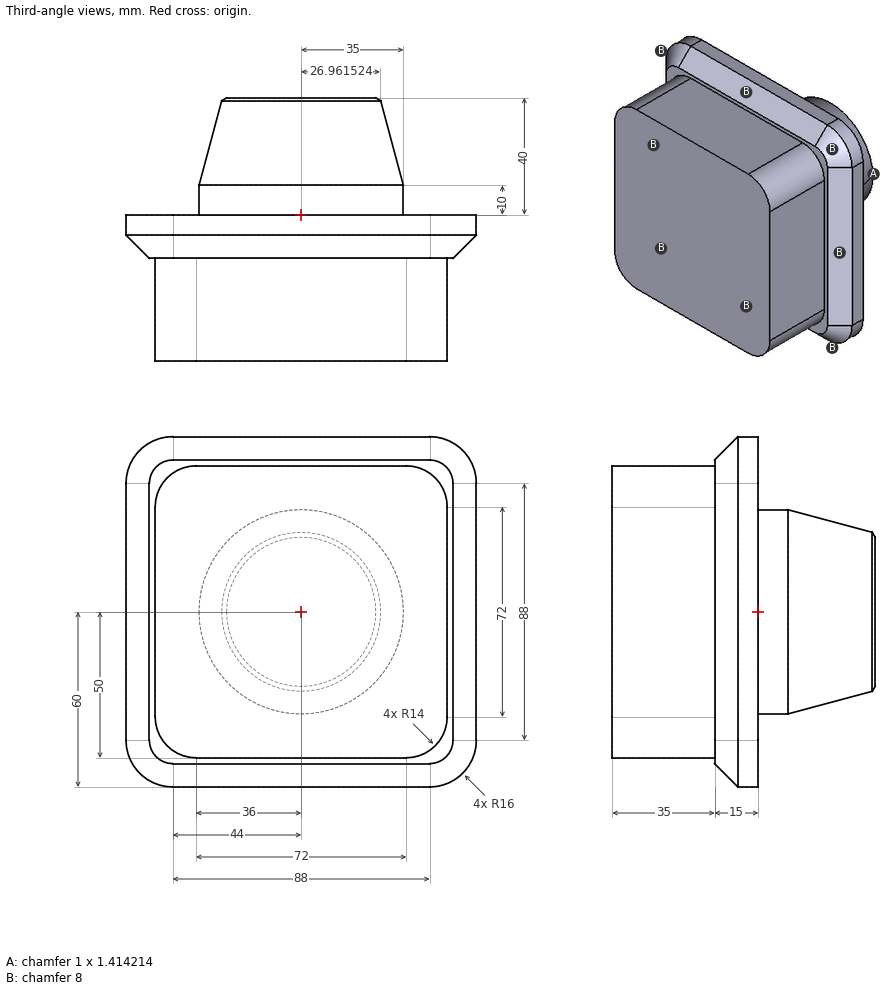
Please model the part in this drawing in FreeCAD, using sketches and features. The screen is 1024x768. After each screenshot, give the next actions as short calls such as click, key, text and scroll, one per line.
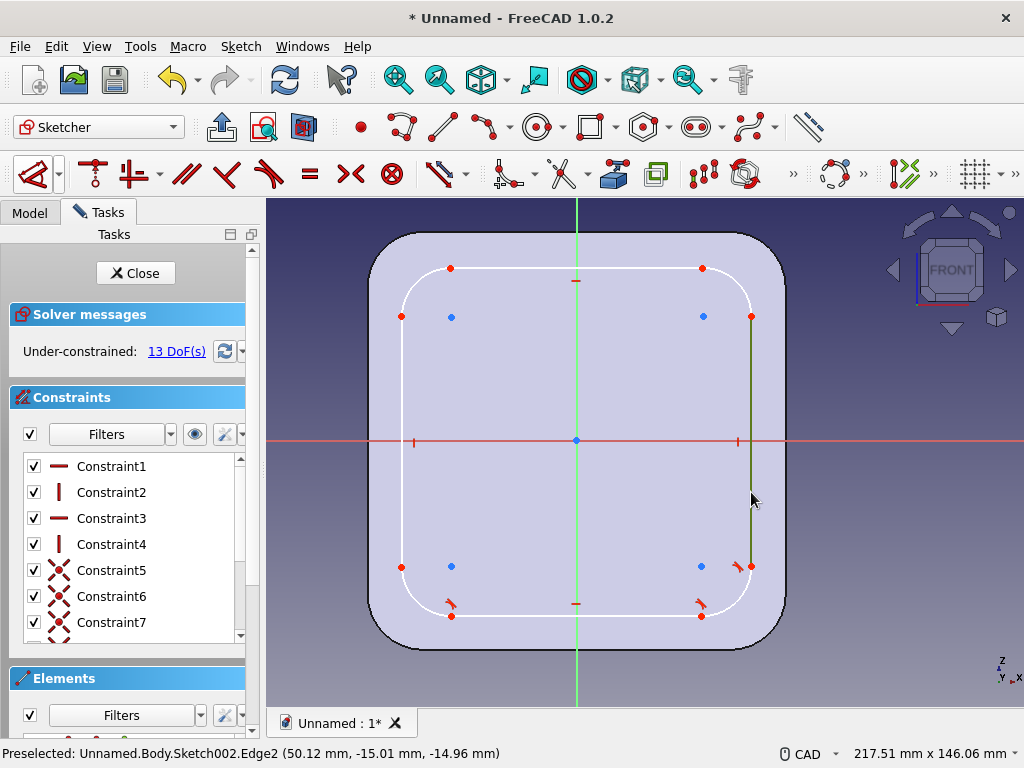
click(746, 295)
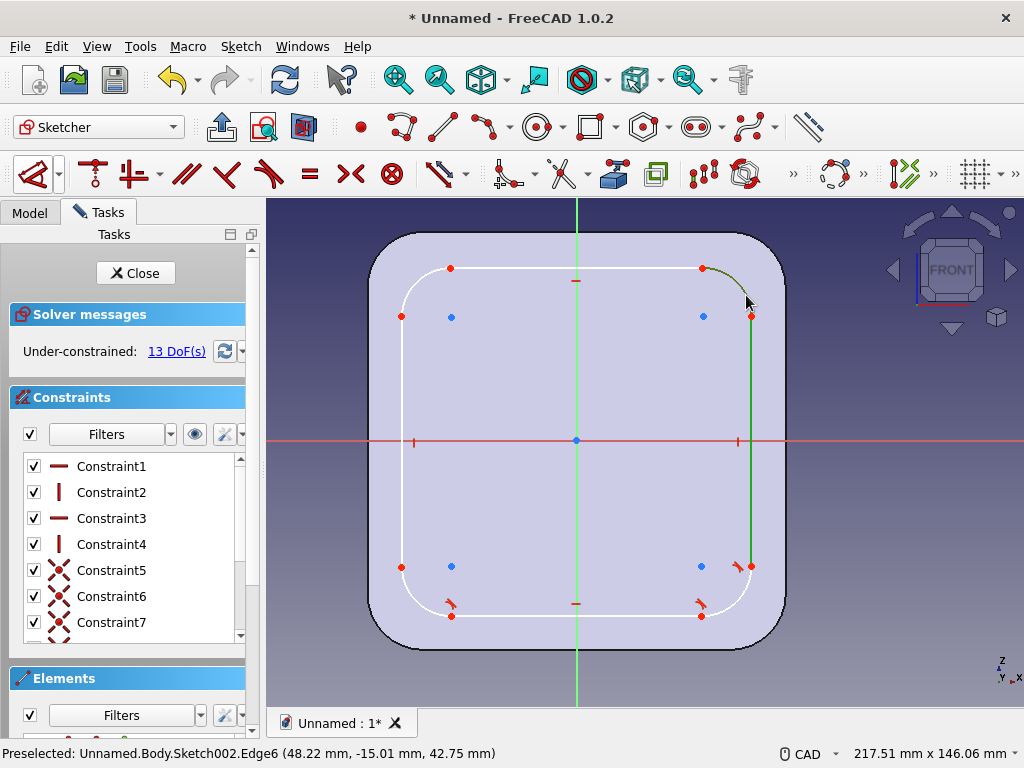
key(t)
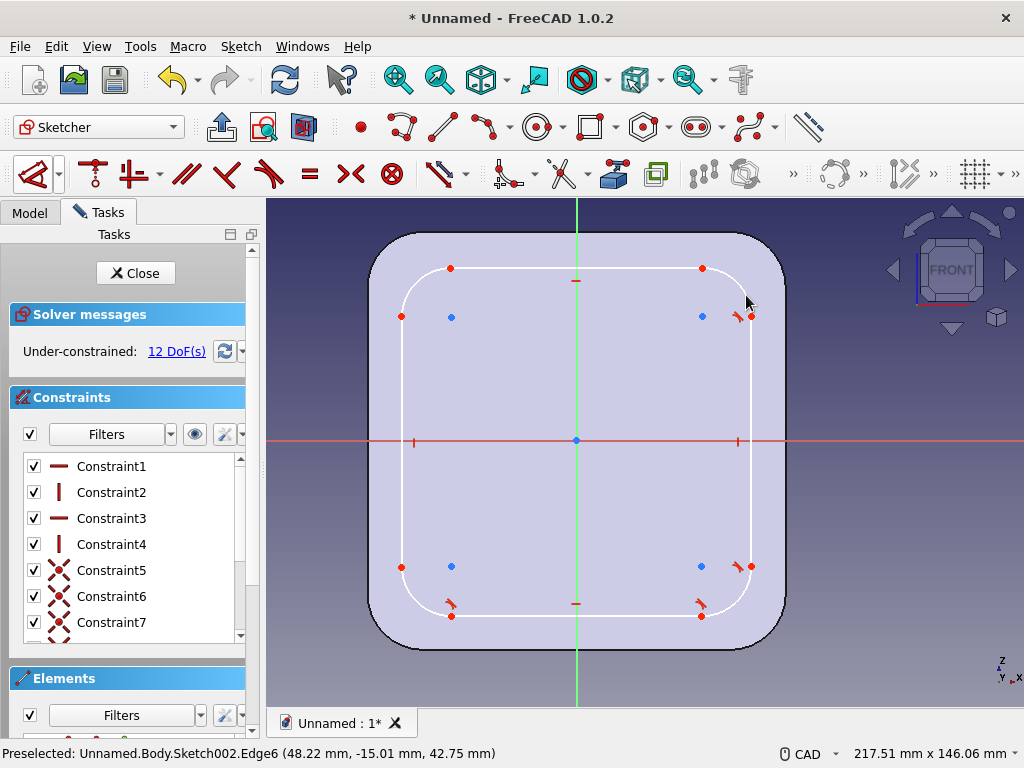
click(627, 268)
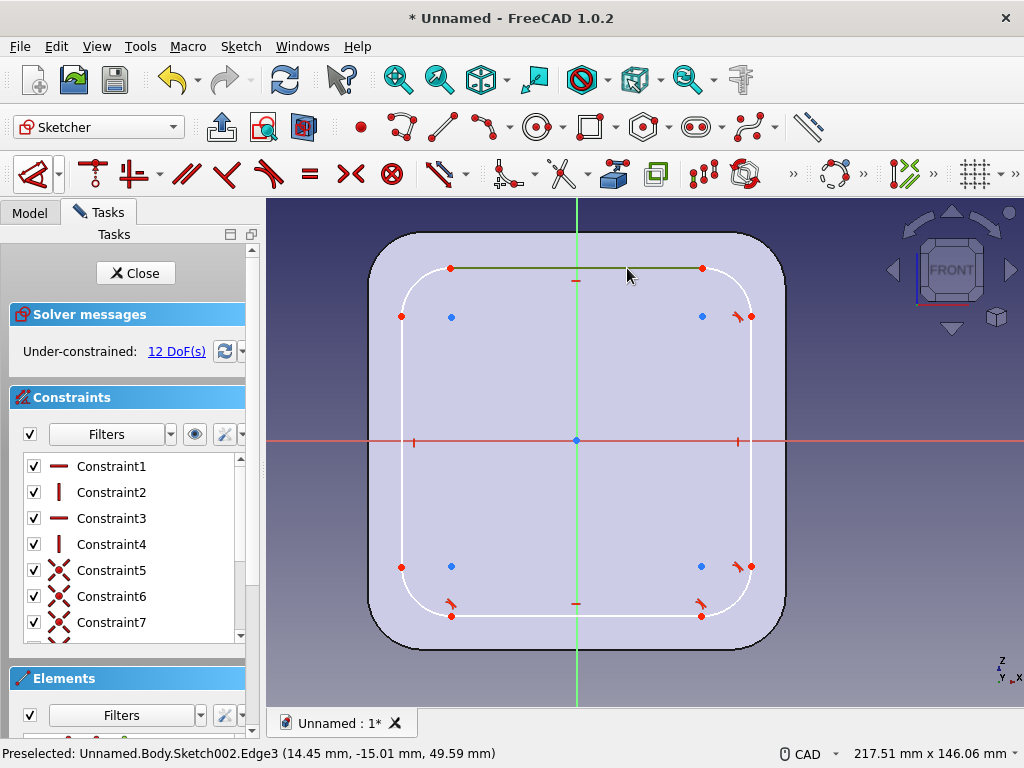
click(746, 295)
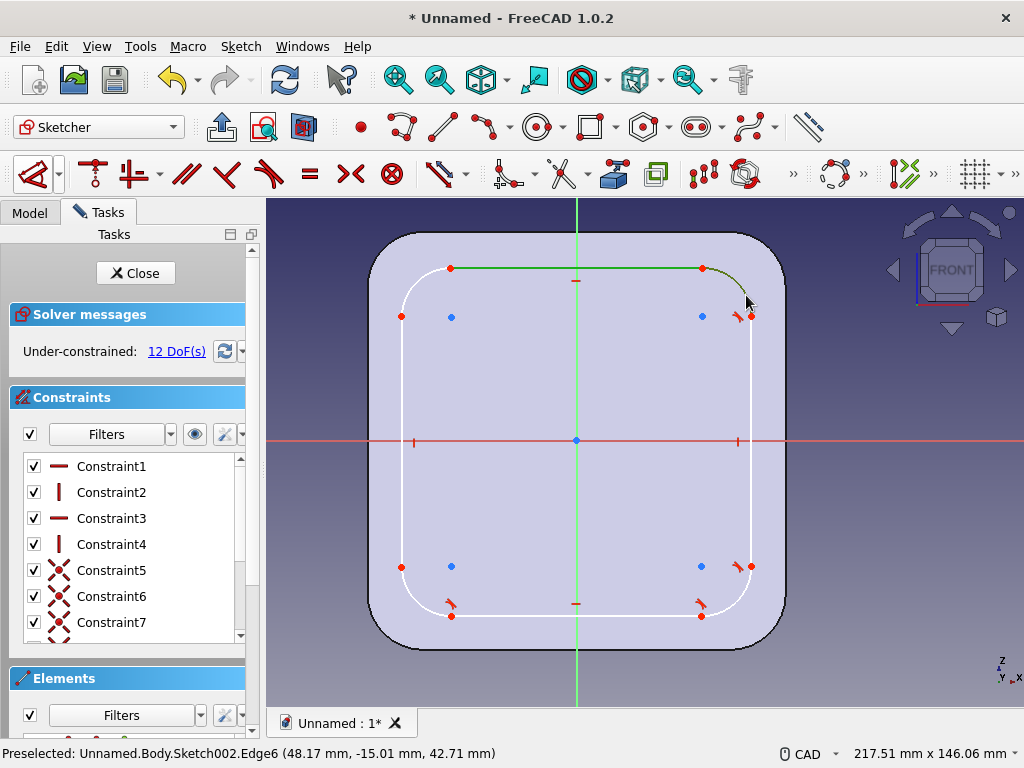
click(269, 174)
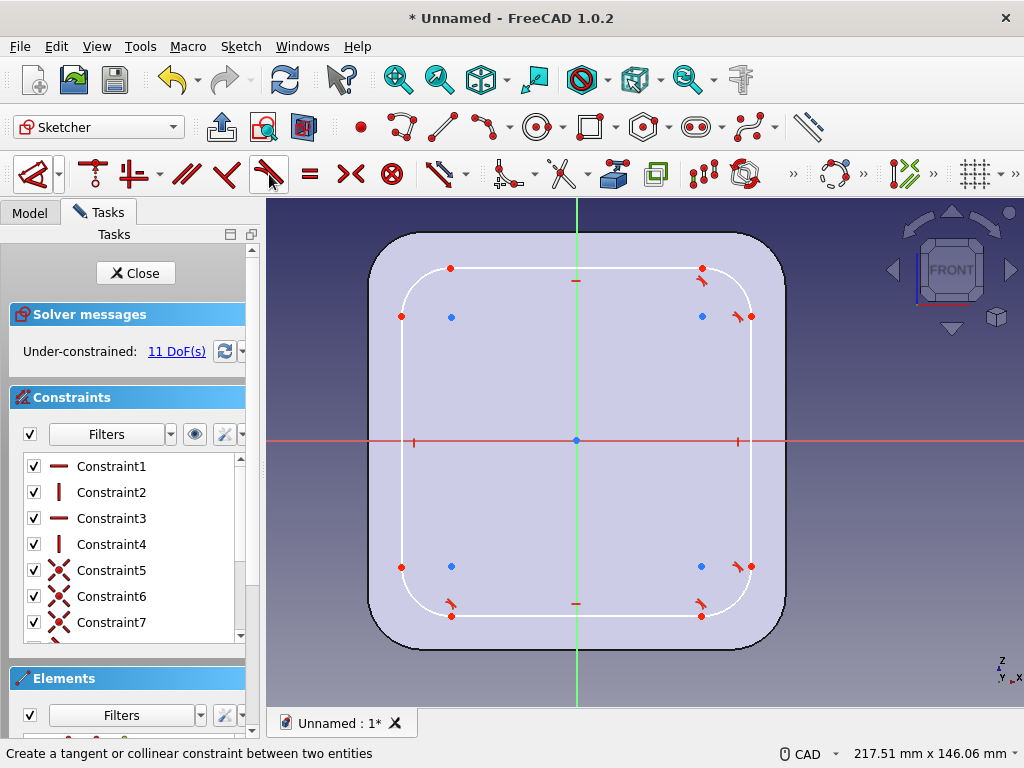
click(627, 268)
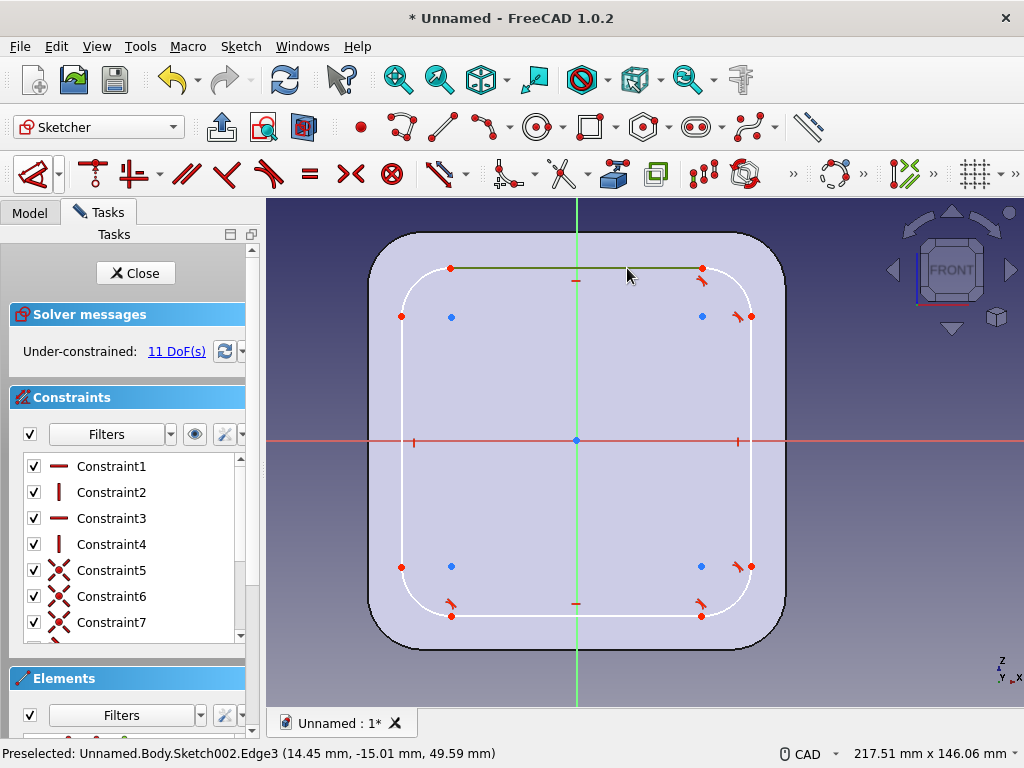
click(429, 274)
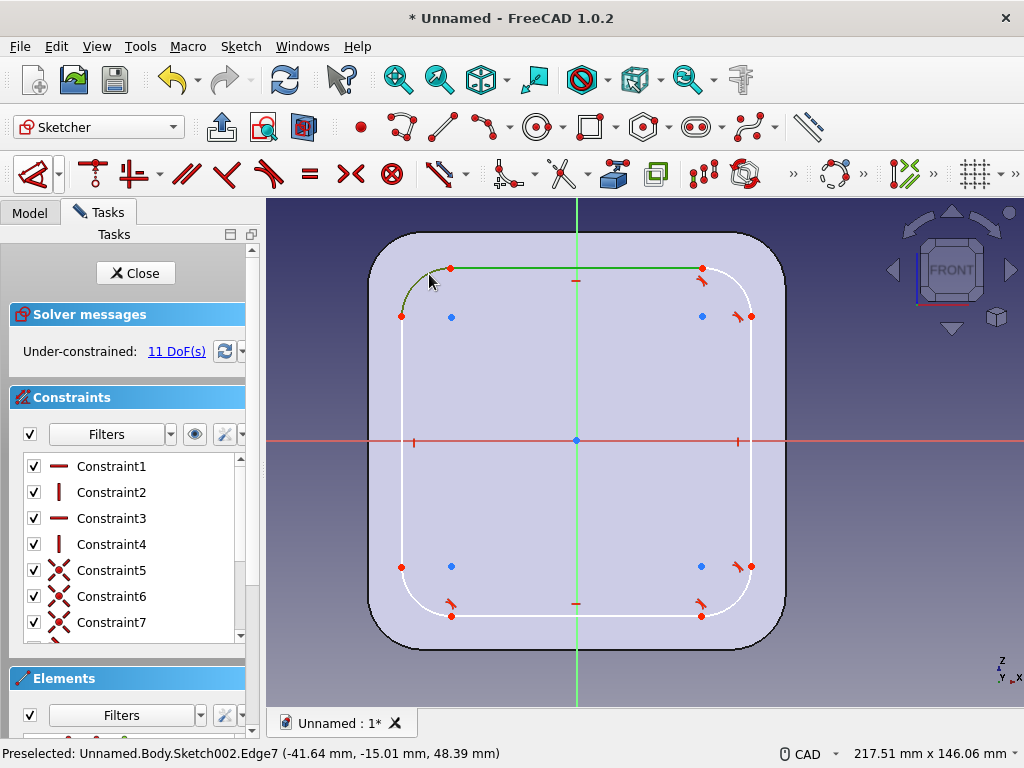
key(t)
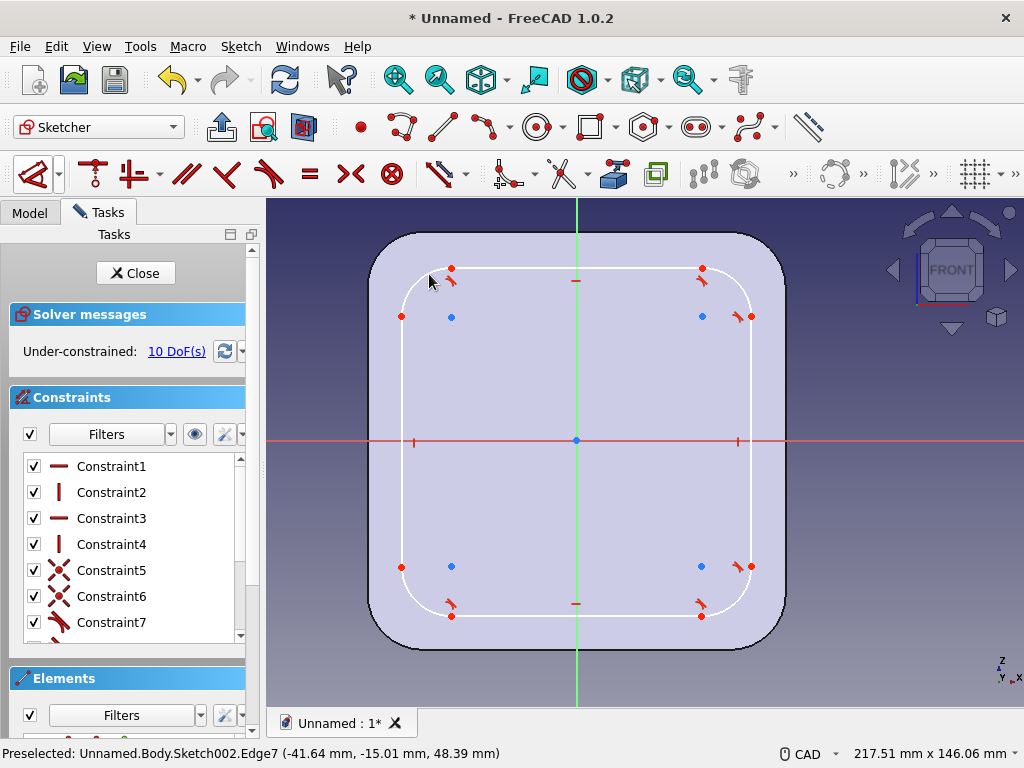
click(402, 392)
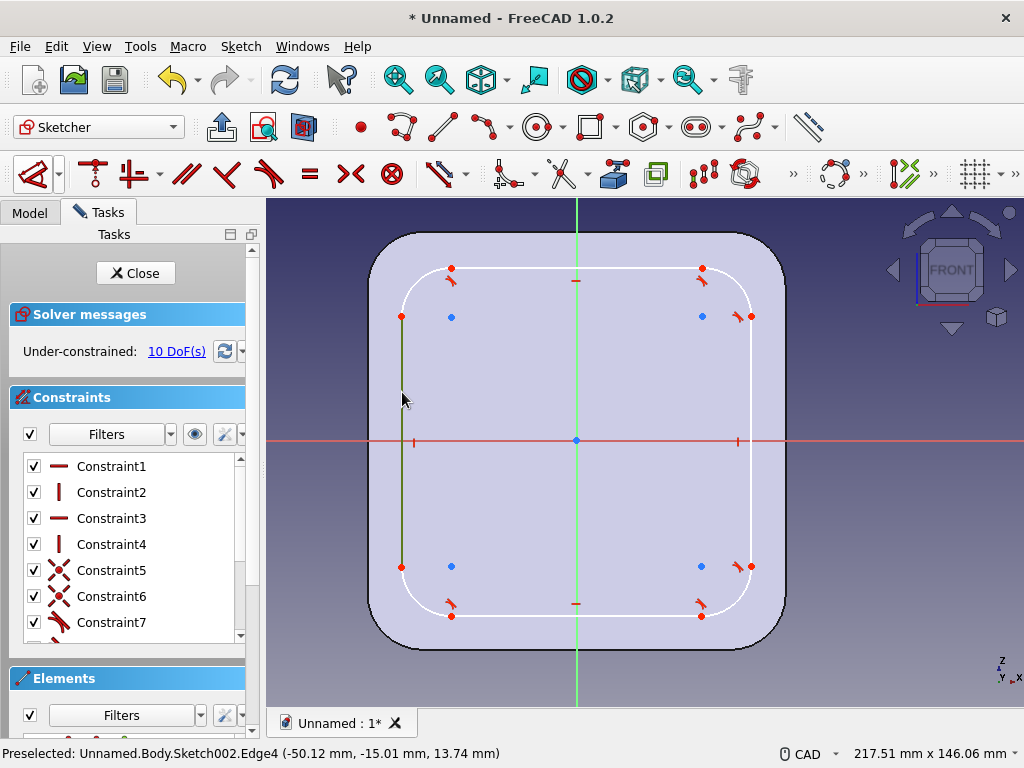
click(429, 273)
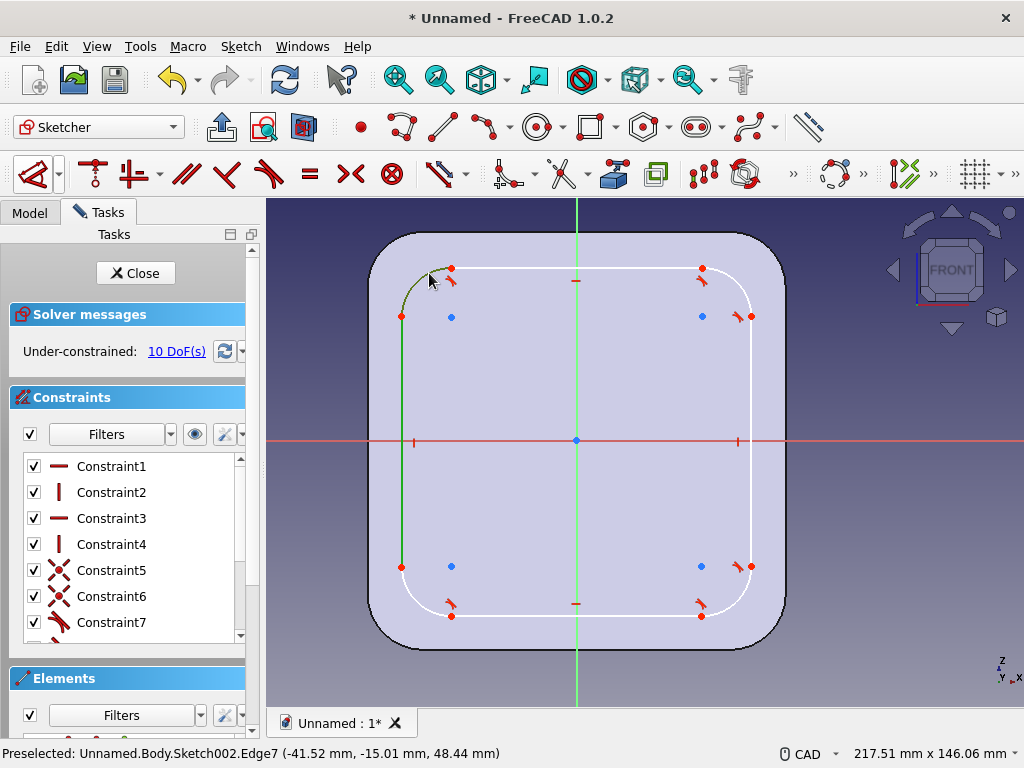
click(269, 174)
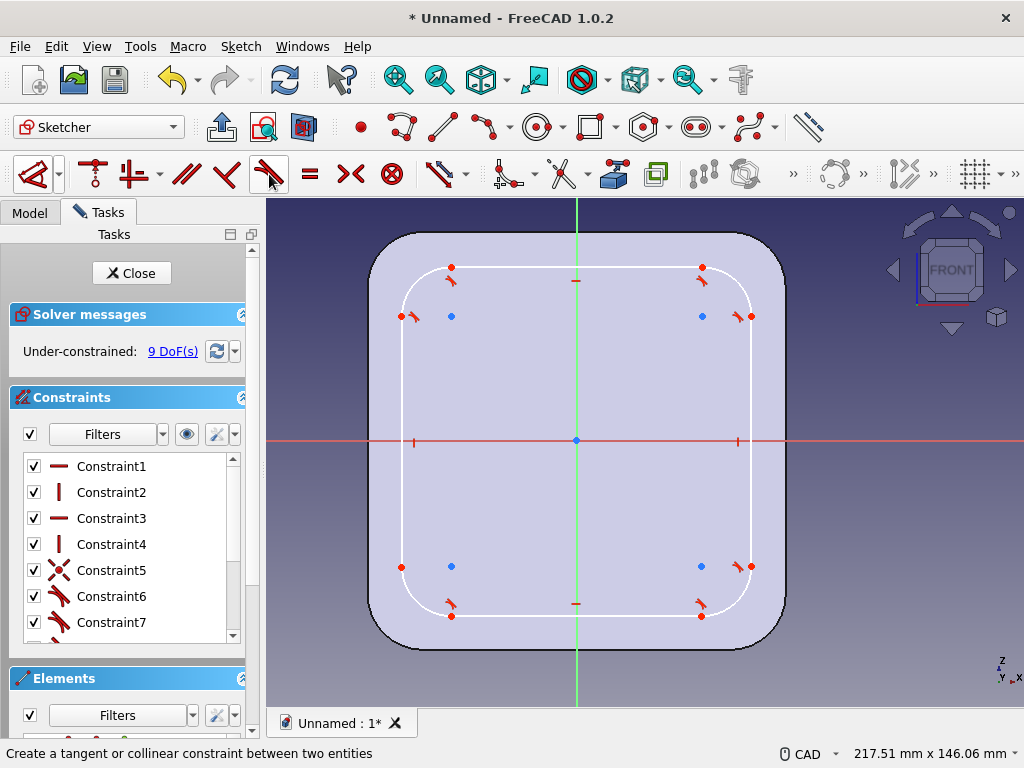
click(402, 392)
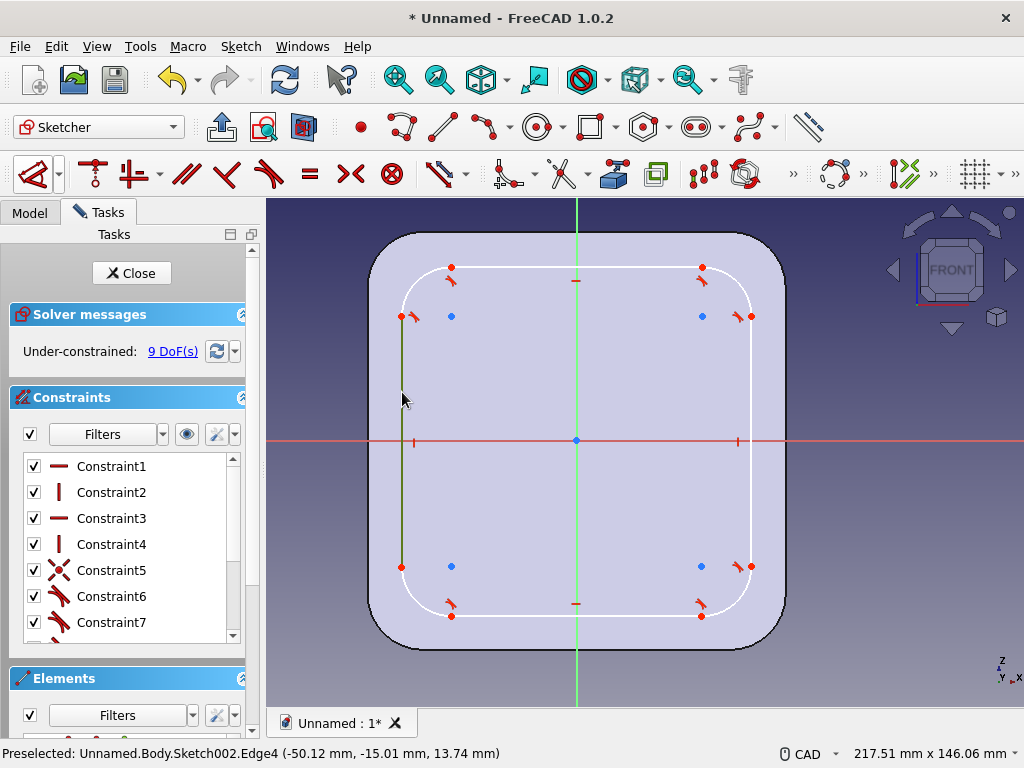
click(408, 590)